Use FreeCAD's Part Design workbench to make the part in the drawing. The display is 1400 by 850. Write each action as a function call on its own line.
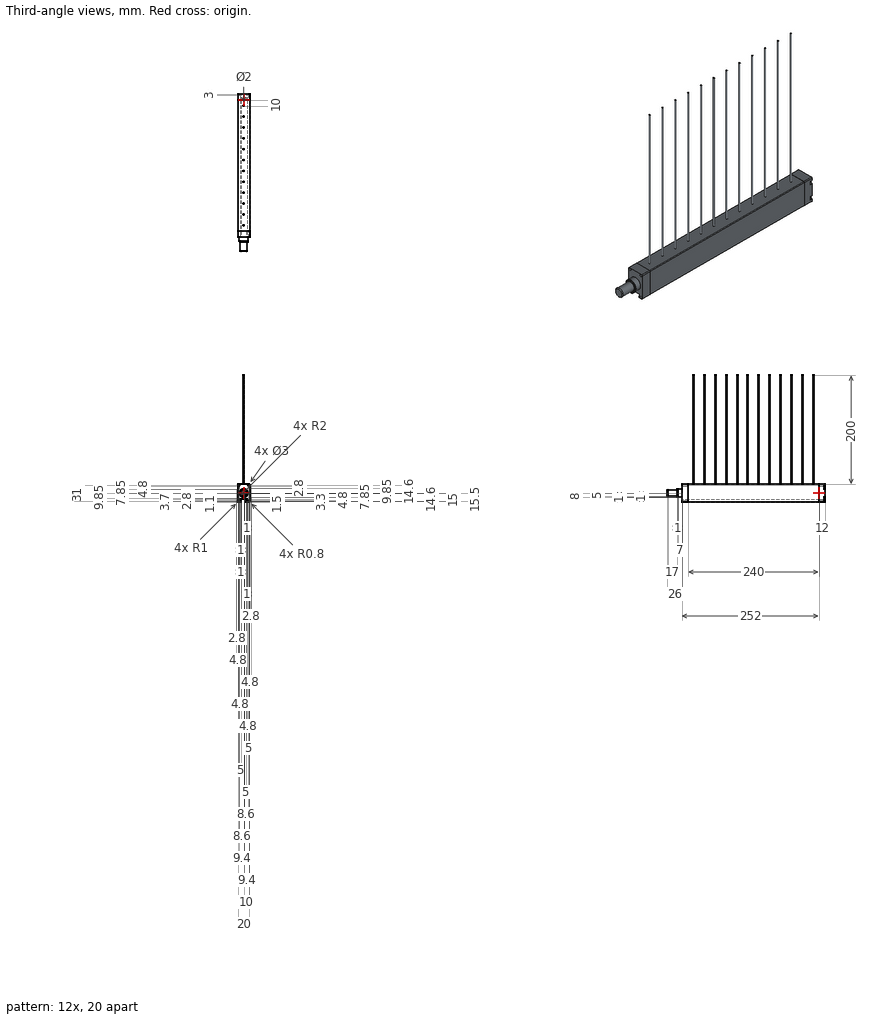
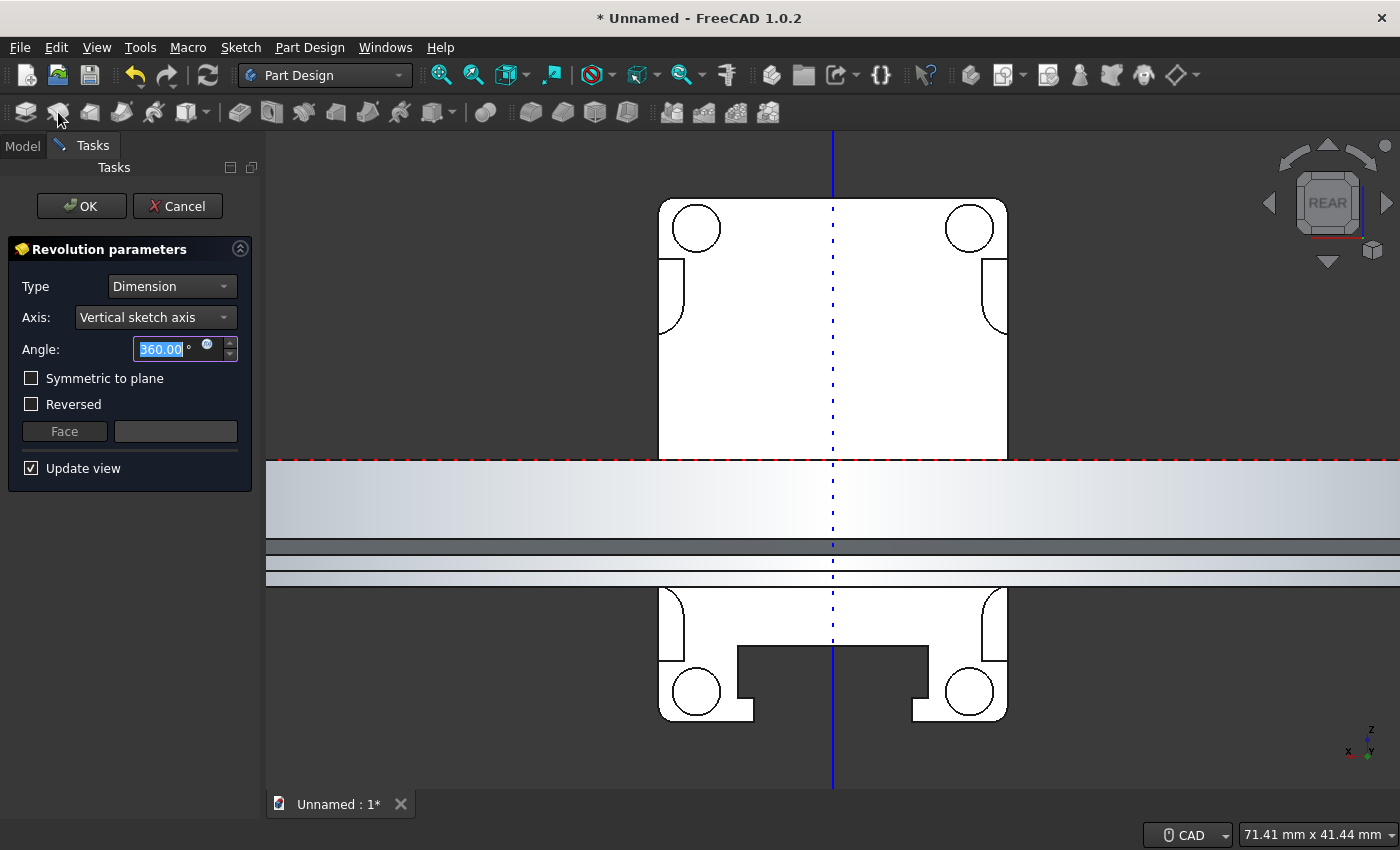
click(156, 318)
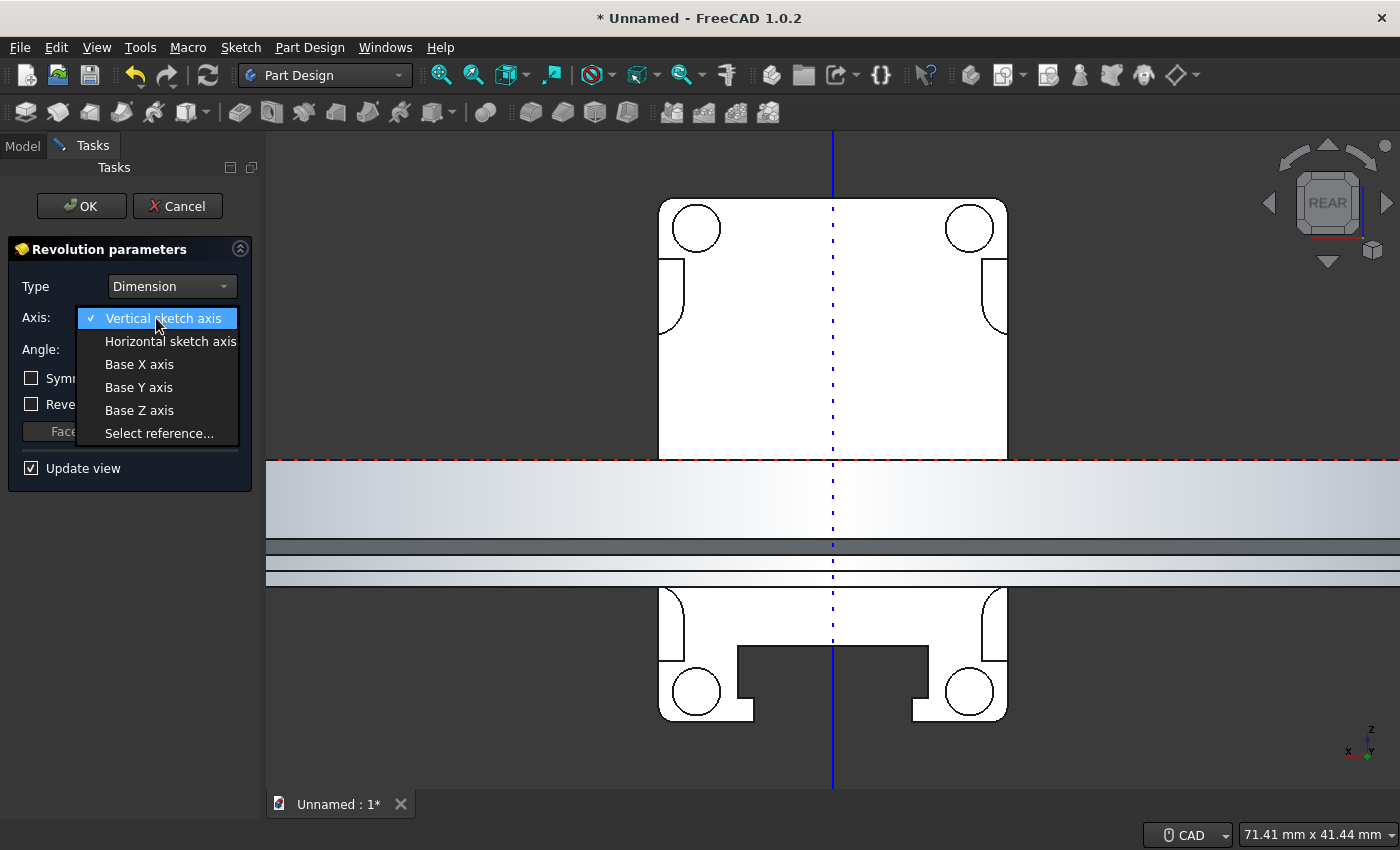
click(156, 342)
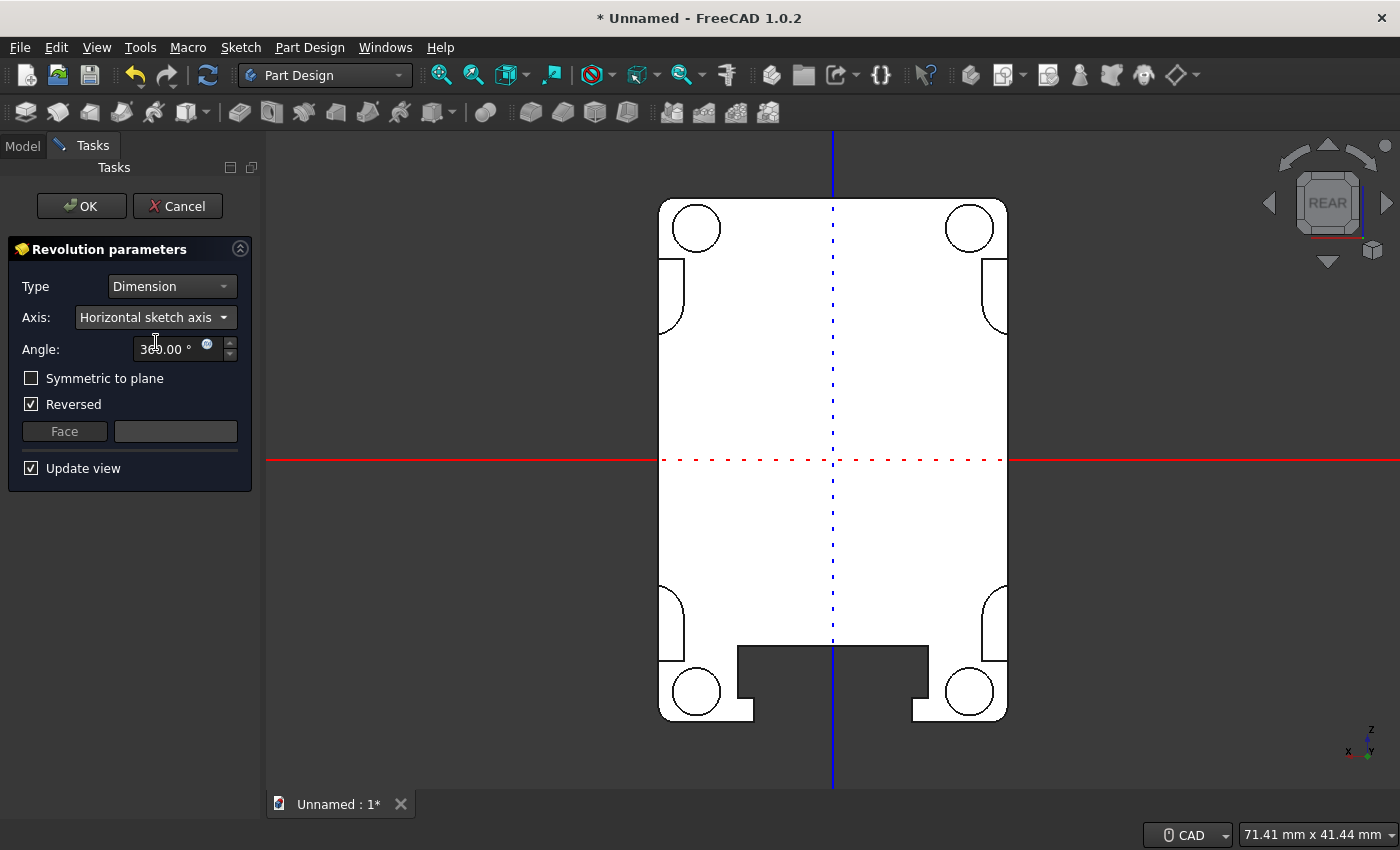
click(82, 206)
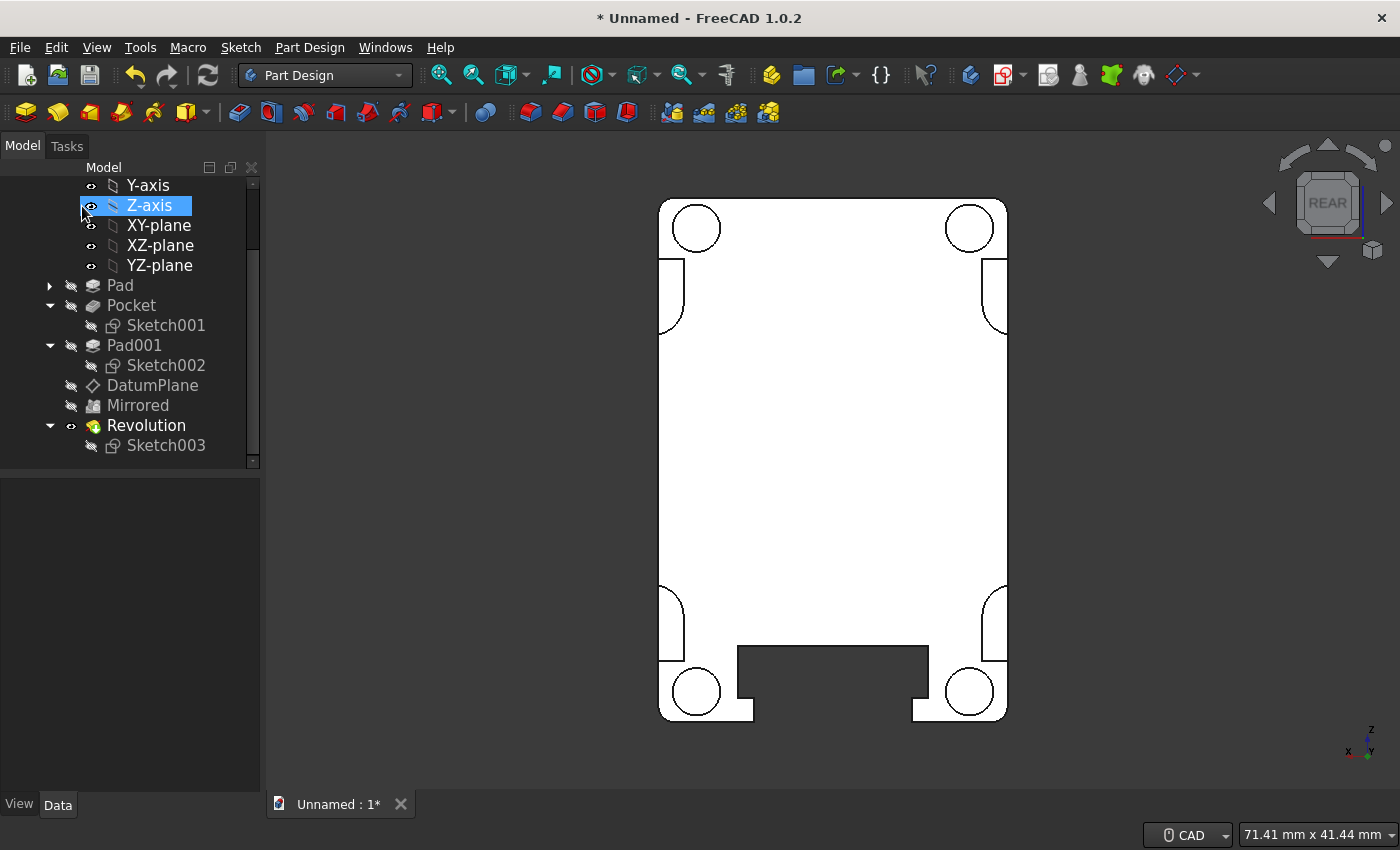
key(0)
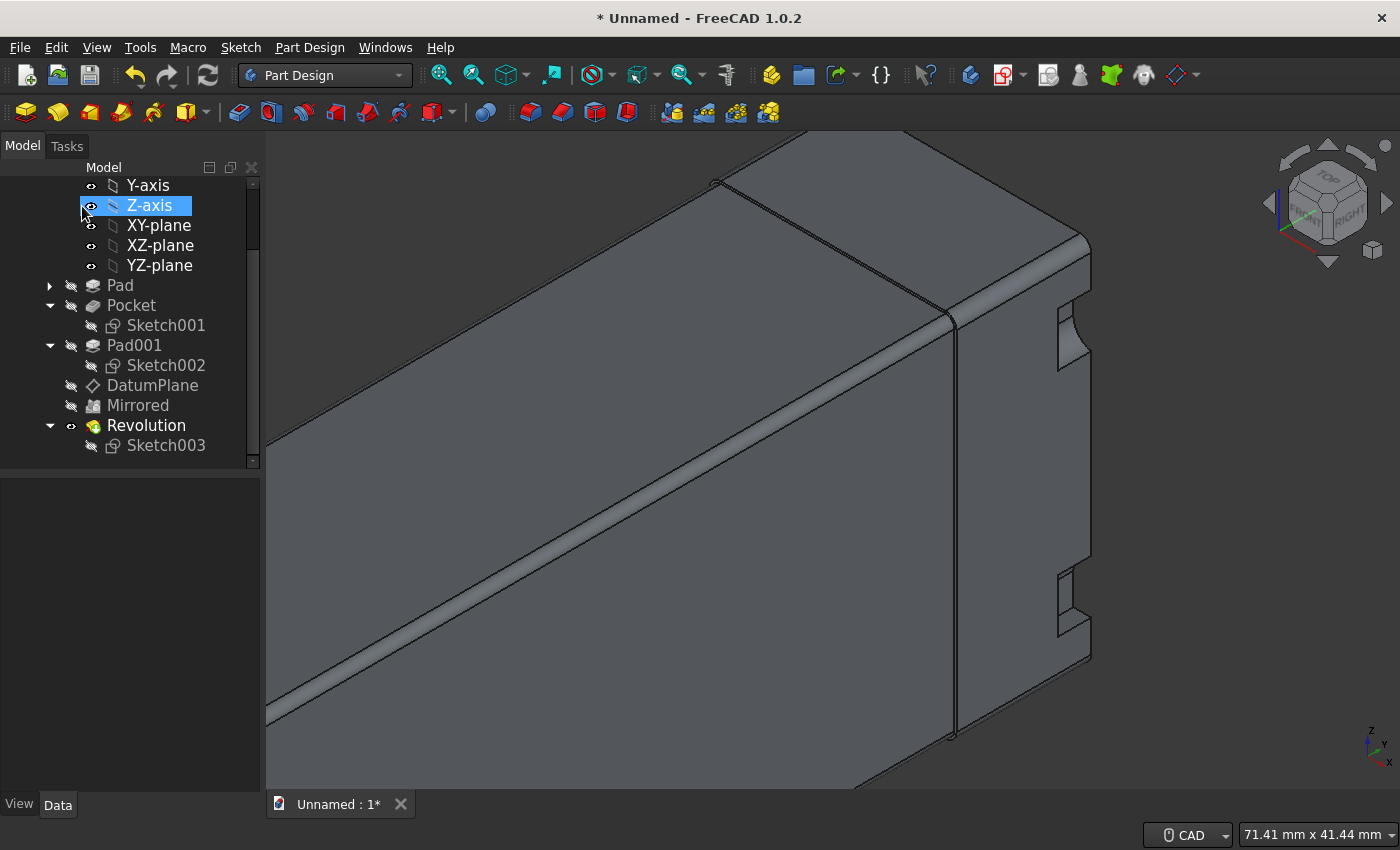
click(442, 76)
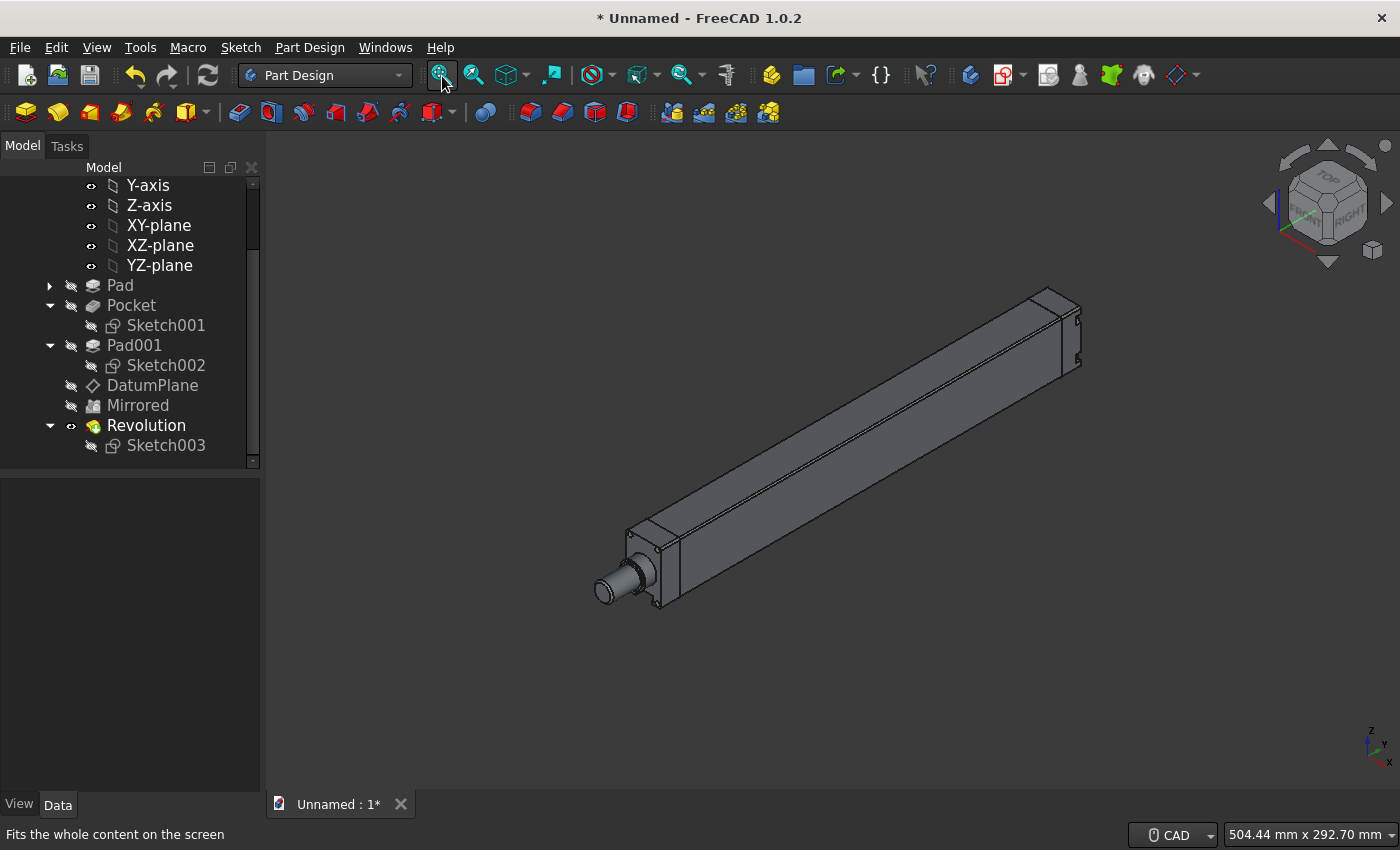
click(1017, 323)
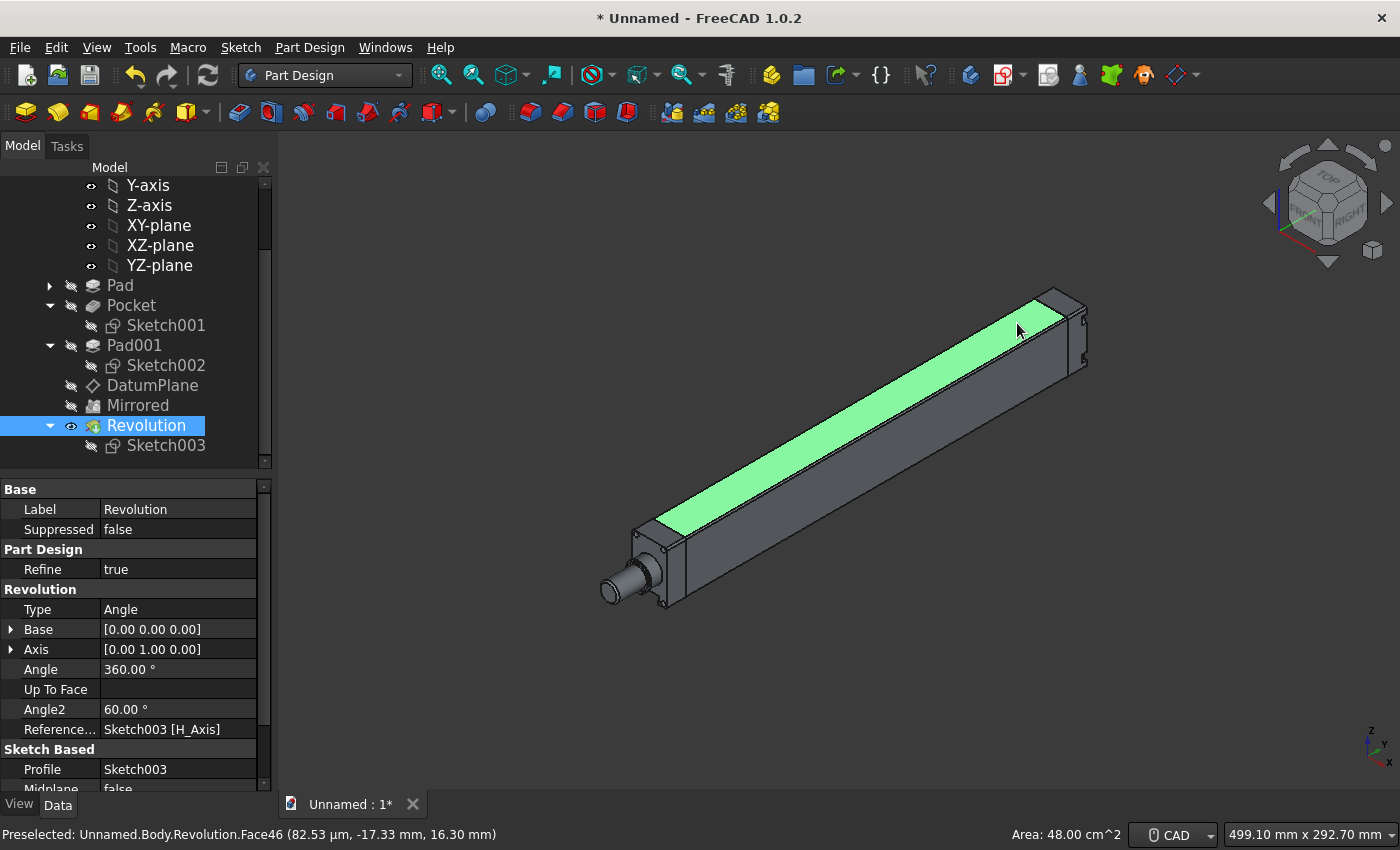
click(1004, 76)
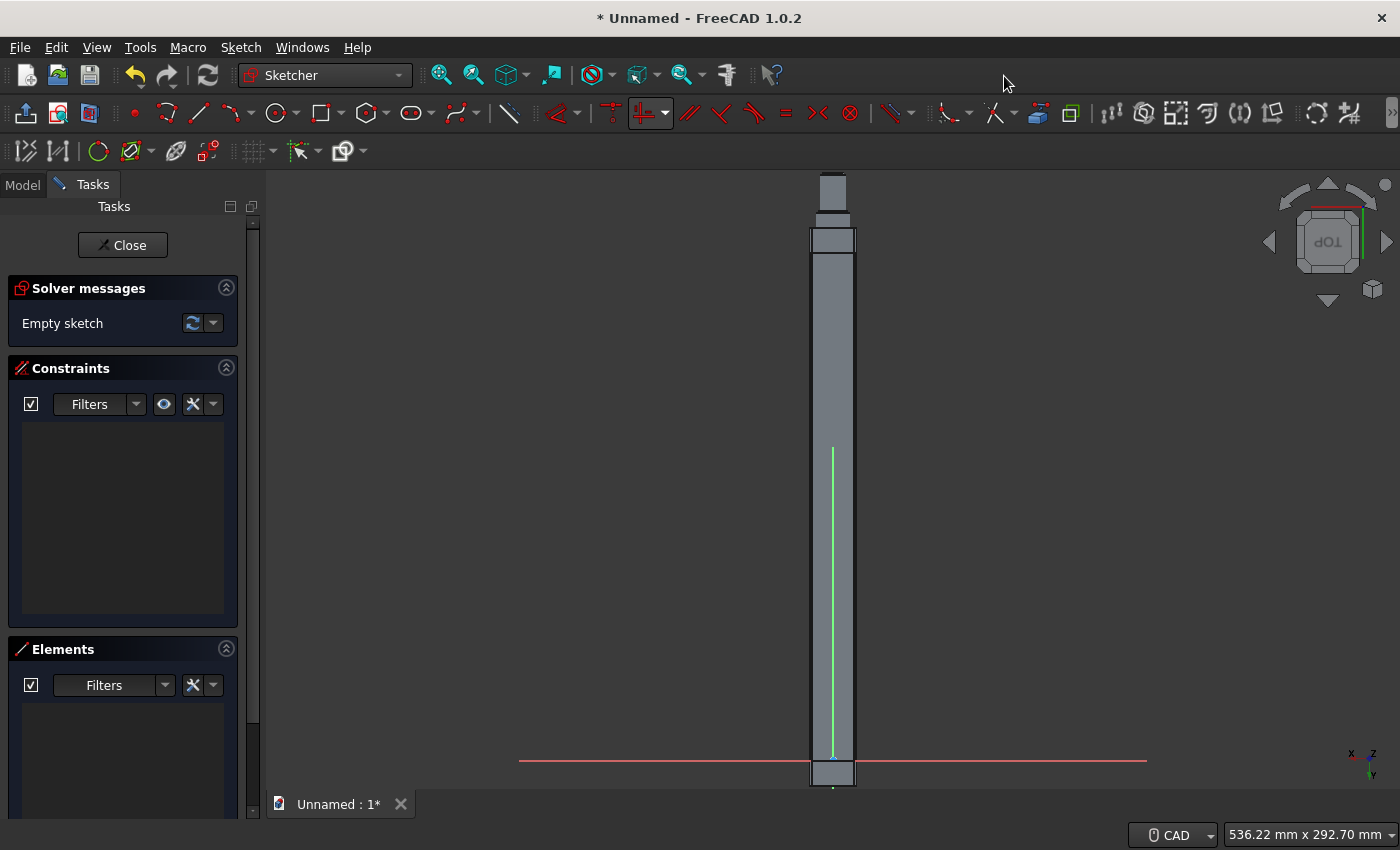
scroll(837, 753, up, 15)